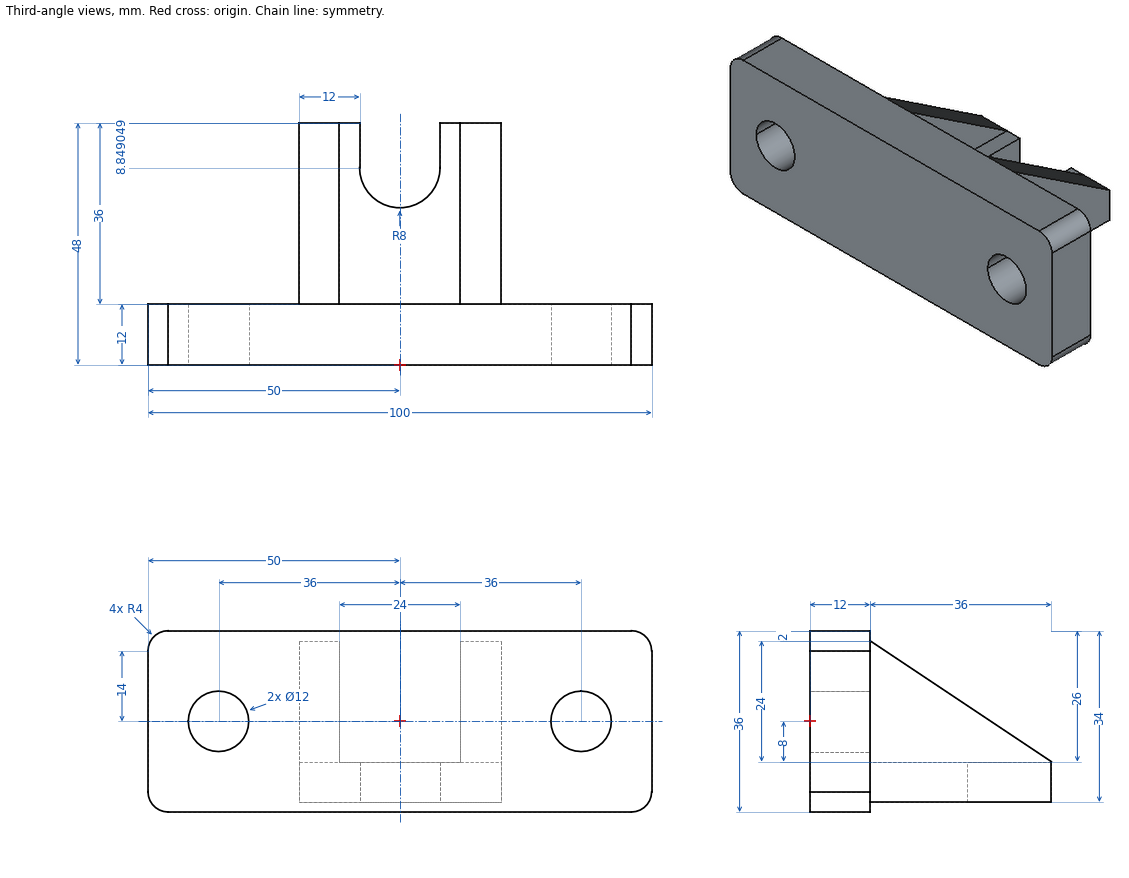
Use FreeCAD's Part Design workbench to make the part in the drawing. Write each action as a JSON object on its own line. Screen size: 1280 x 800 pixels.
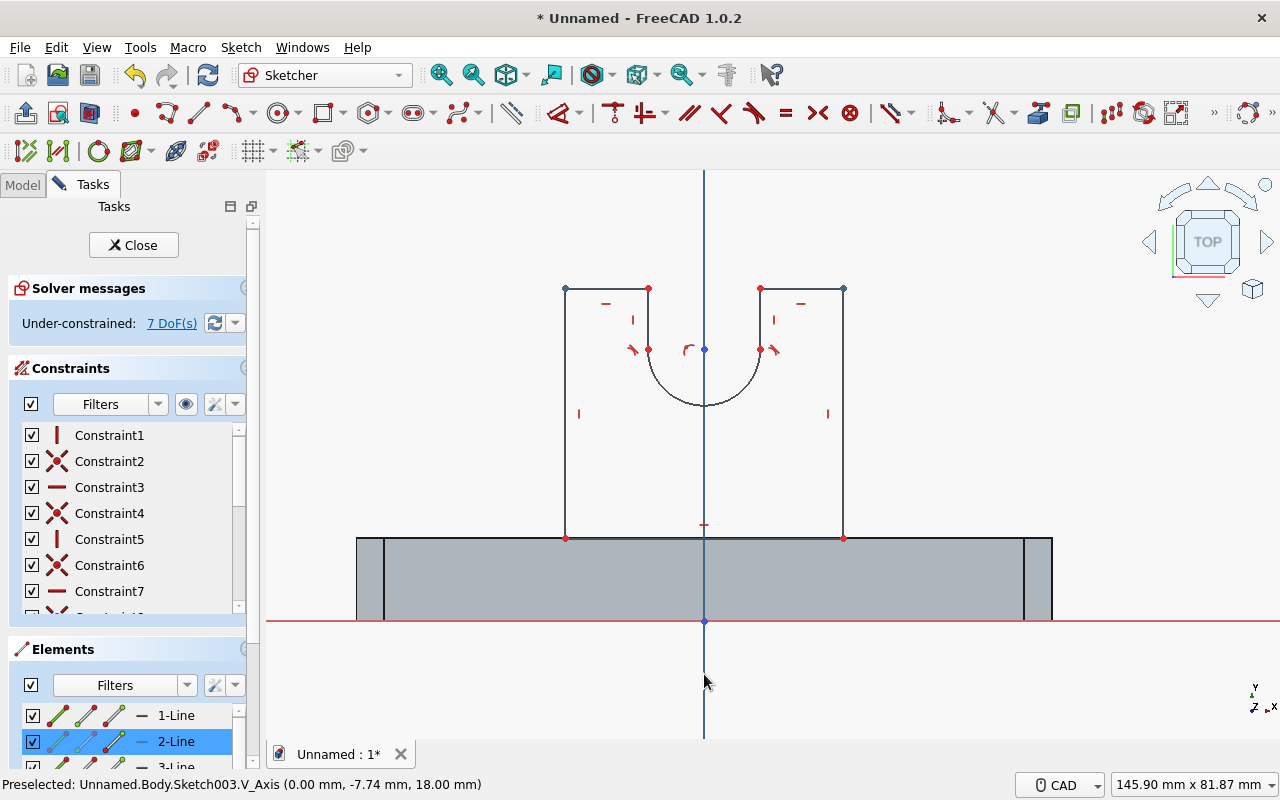
{"action": "left_click", "coordinate": [818, 114]}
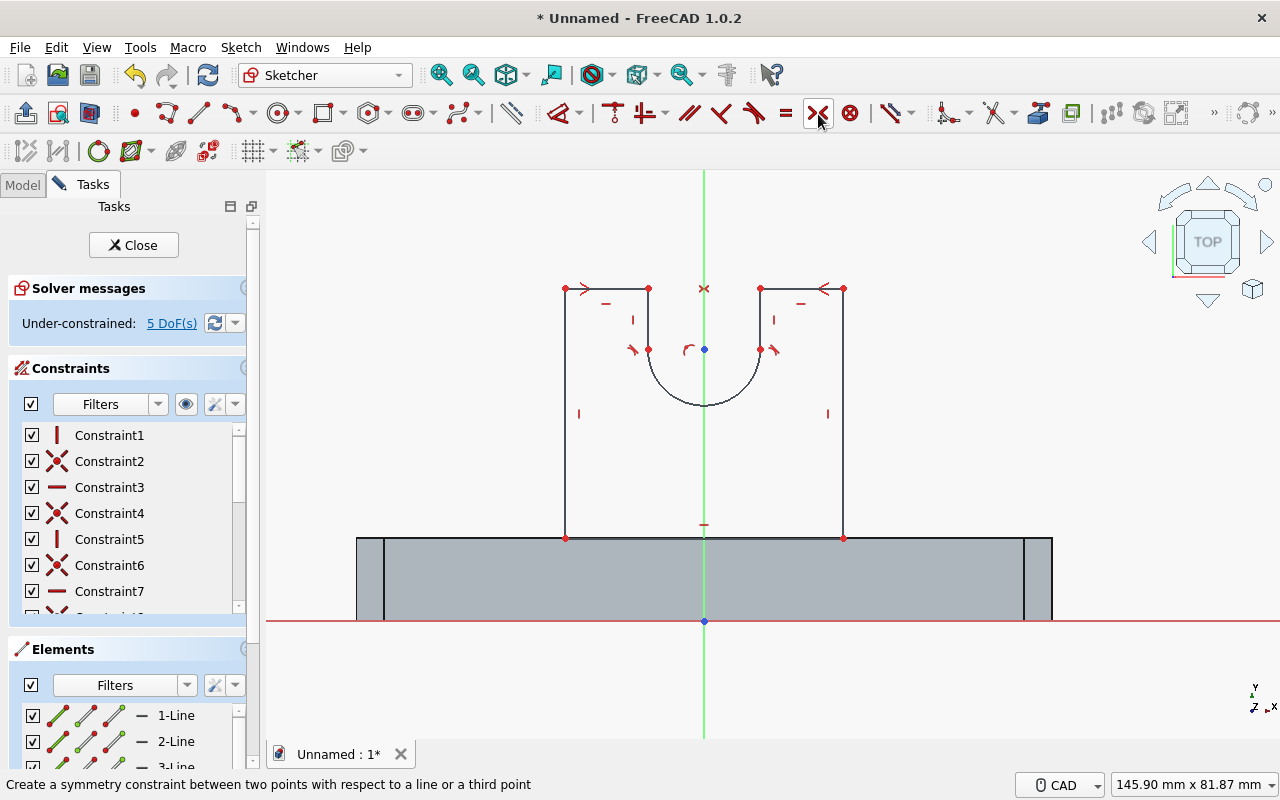
{"action": "left_click", "coordinate": [558, 114]}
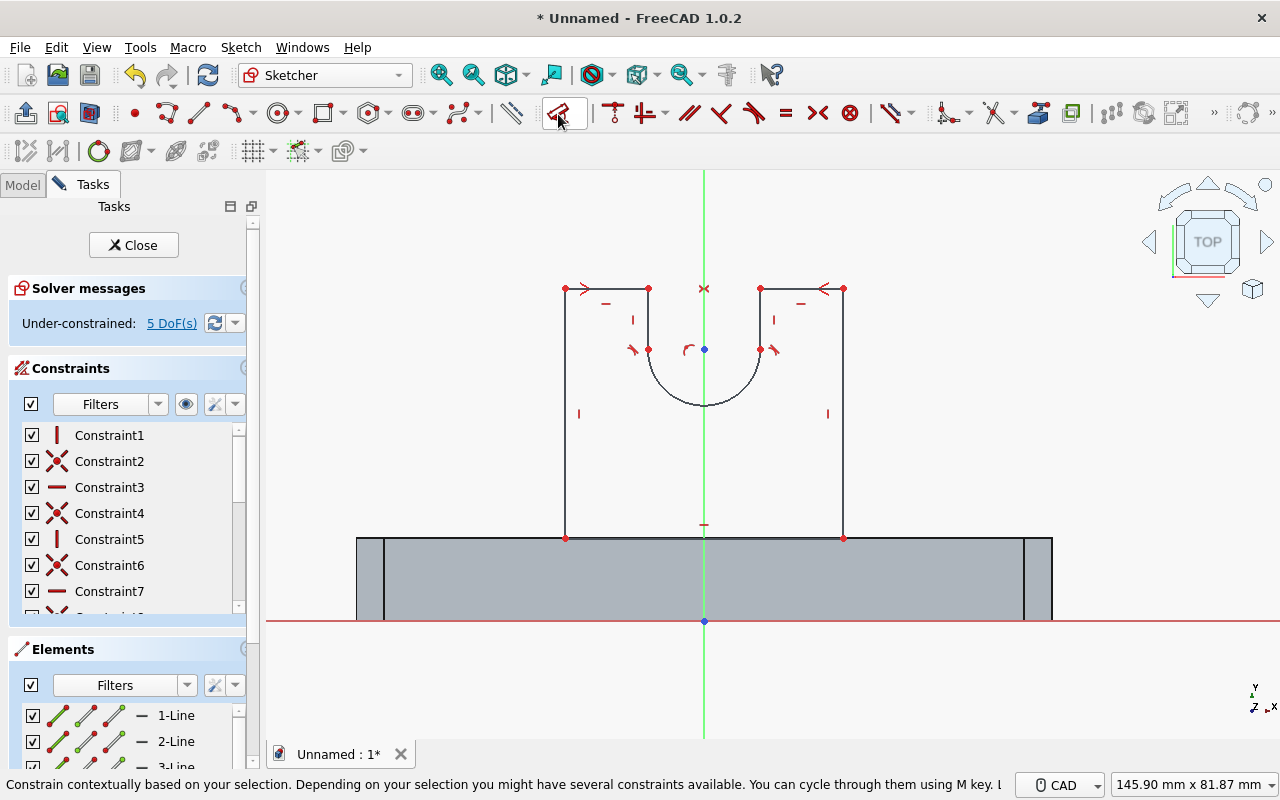
{"action": "left_click", "coordinate": [671, 395]}
{"action": "left_click", "coordinate": [652, 421]}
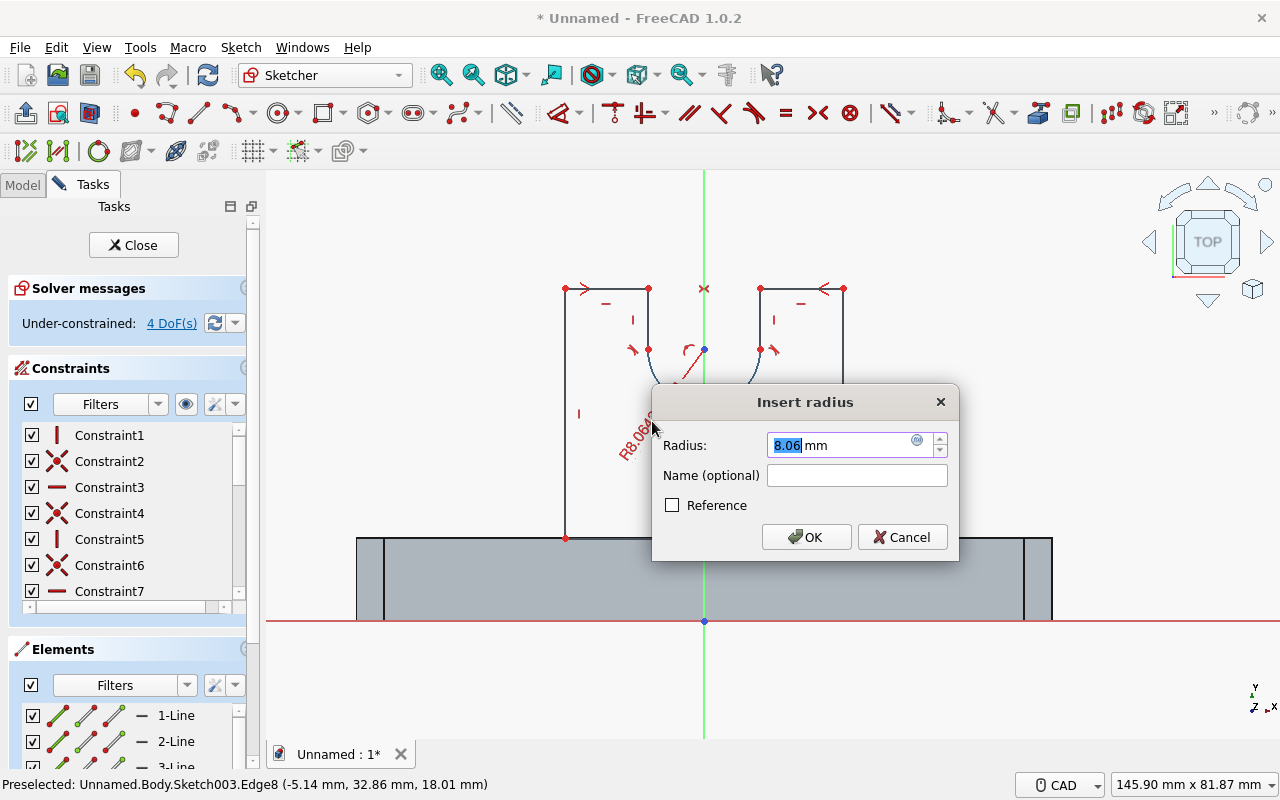
{"action": "type", "text": "8"}
{"action": "key", "text": "Return"}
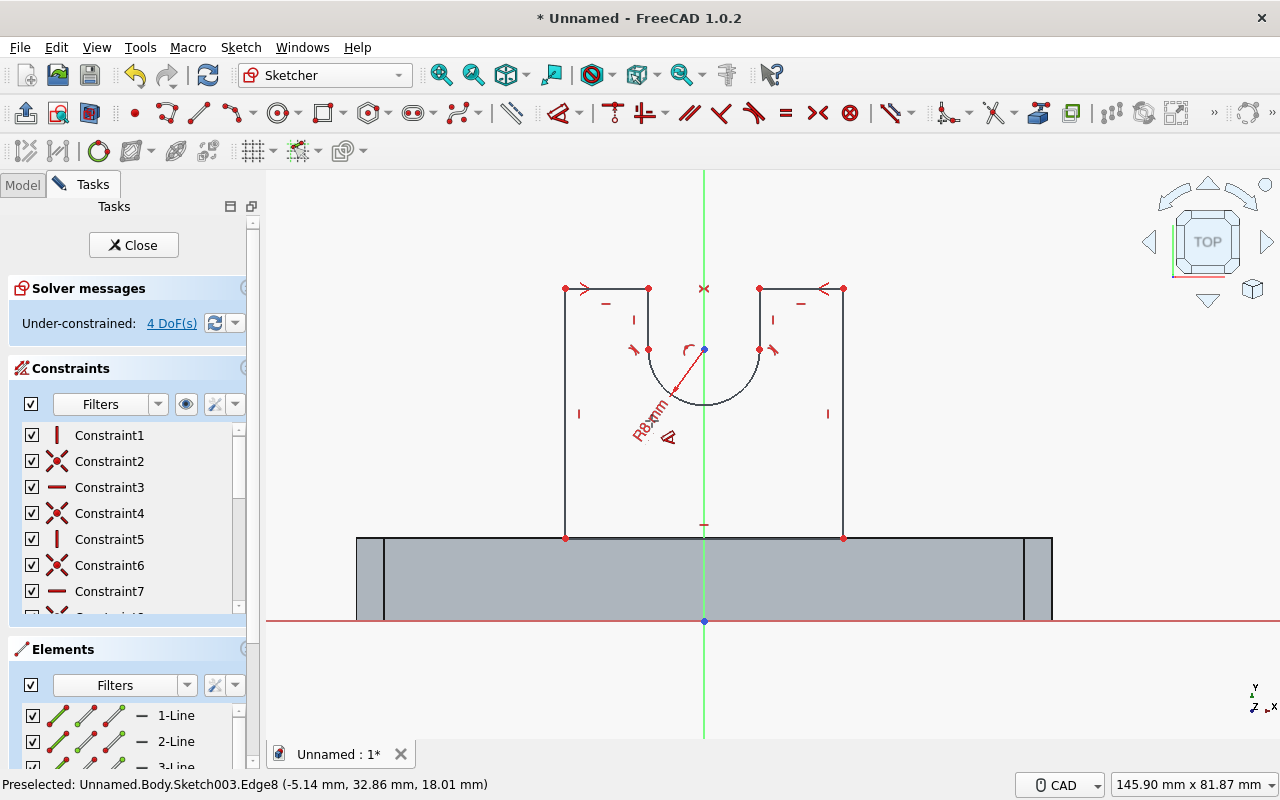
{"action": "left_click", "coordinate": [623, 289]}
{"action": "left_click", "coordinate": [607, 255]}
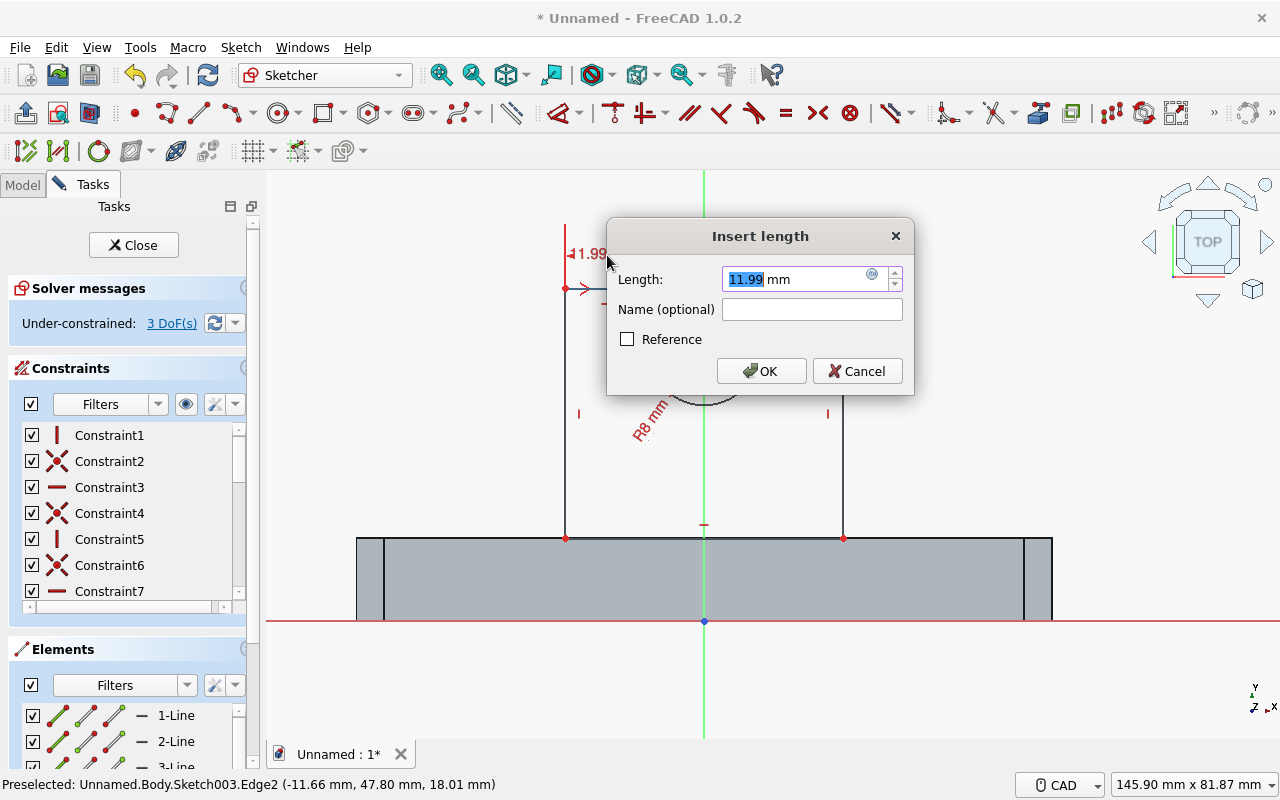
{"action": "type", "text": "12"}
{"action": "key", "text": "Return"}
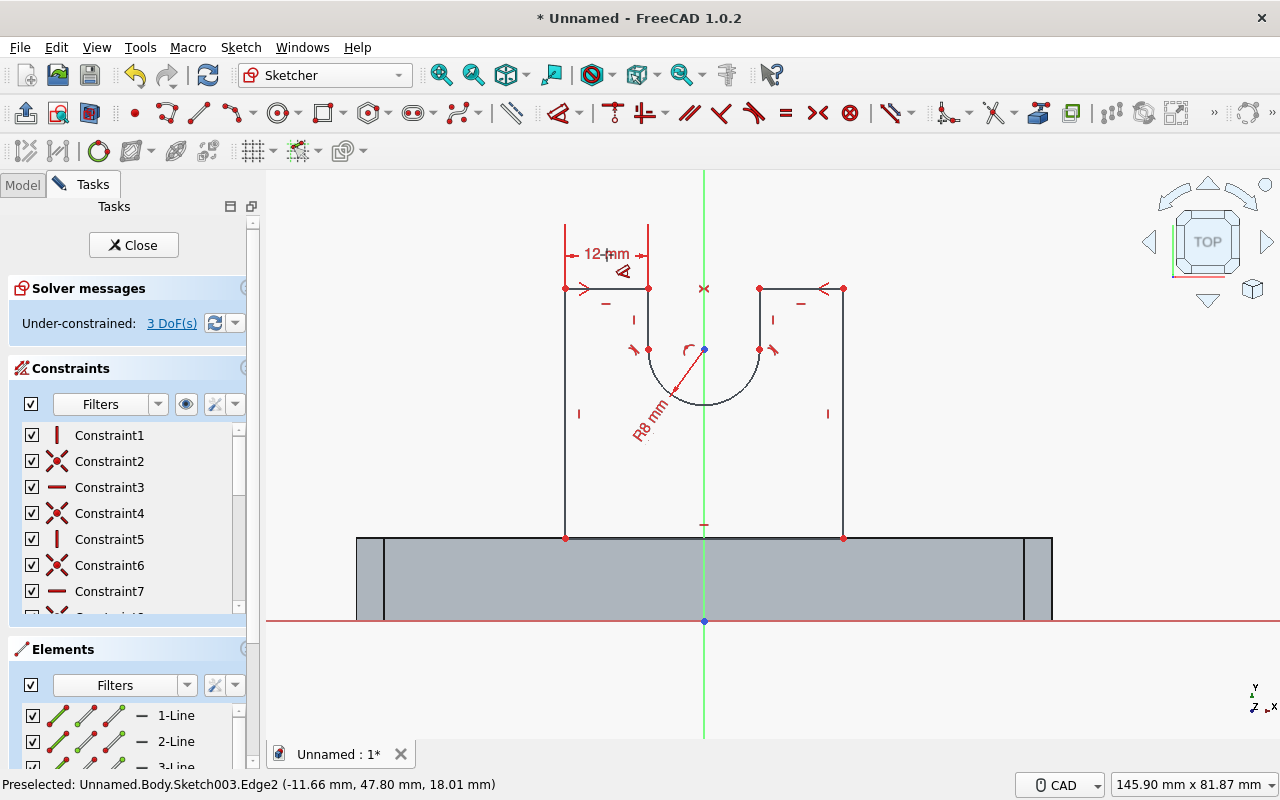
{"action": "left_click", "coordinate": [565, 364]}
{"action": "left_click", "coordinate": [531, 414]}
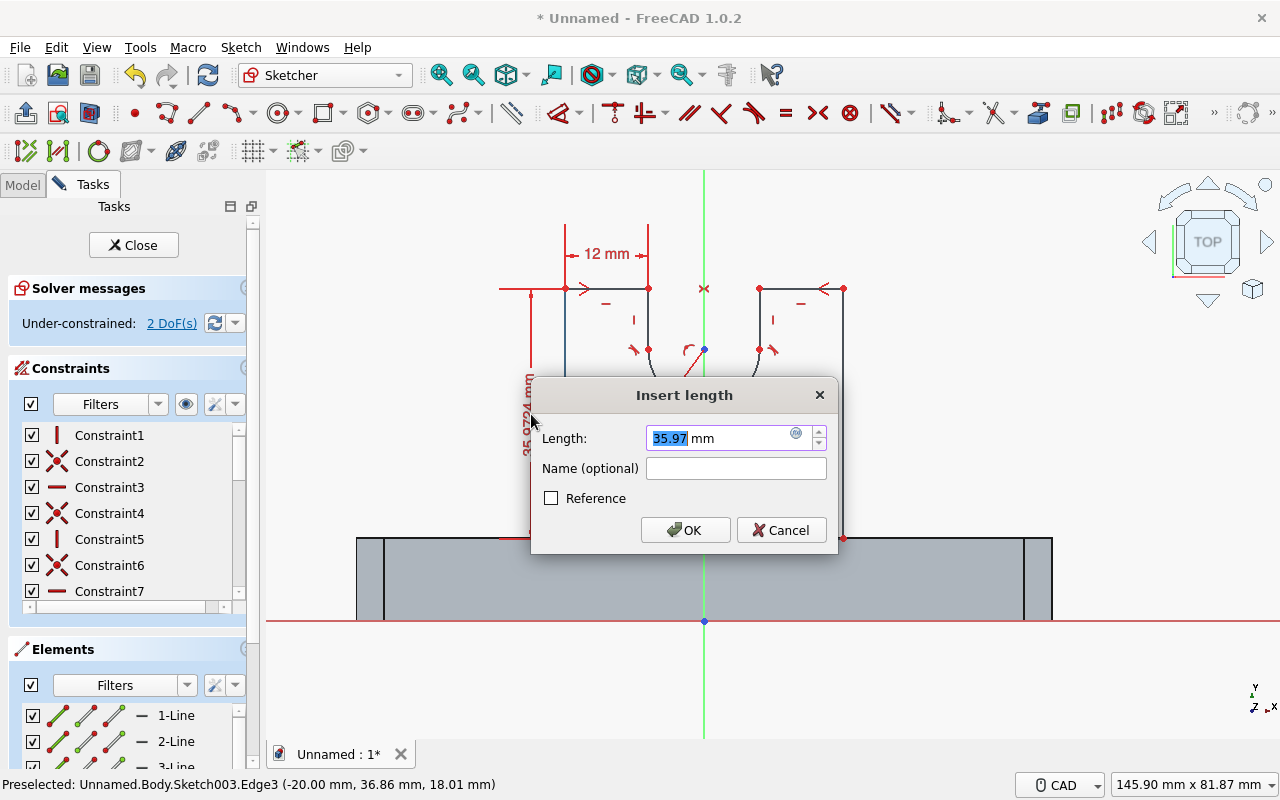
{"action": "type", "text": "36"}
{"action": "key", "text": "Return"}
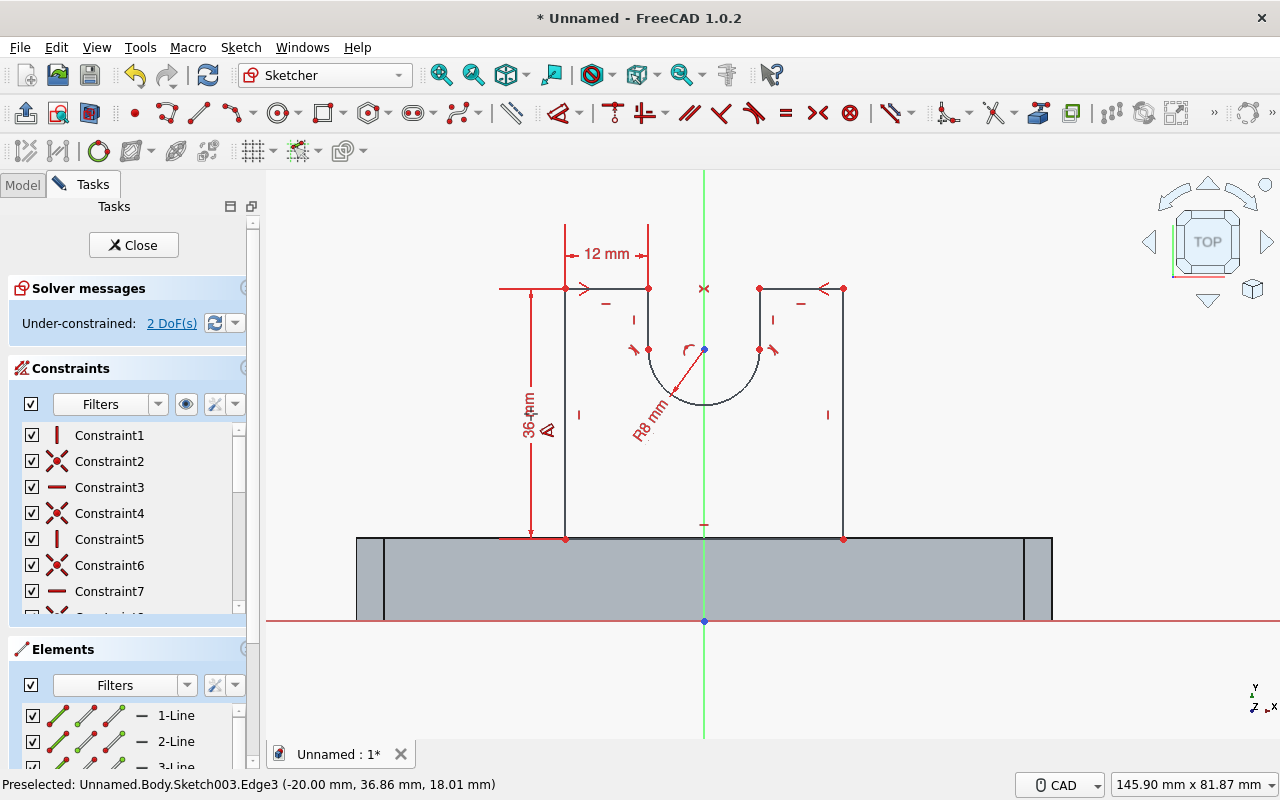
{"action": "left_click", "coordinate": [648, 289]}
{"action": "left_click", "coordinate": [614, 455]}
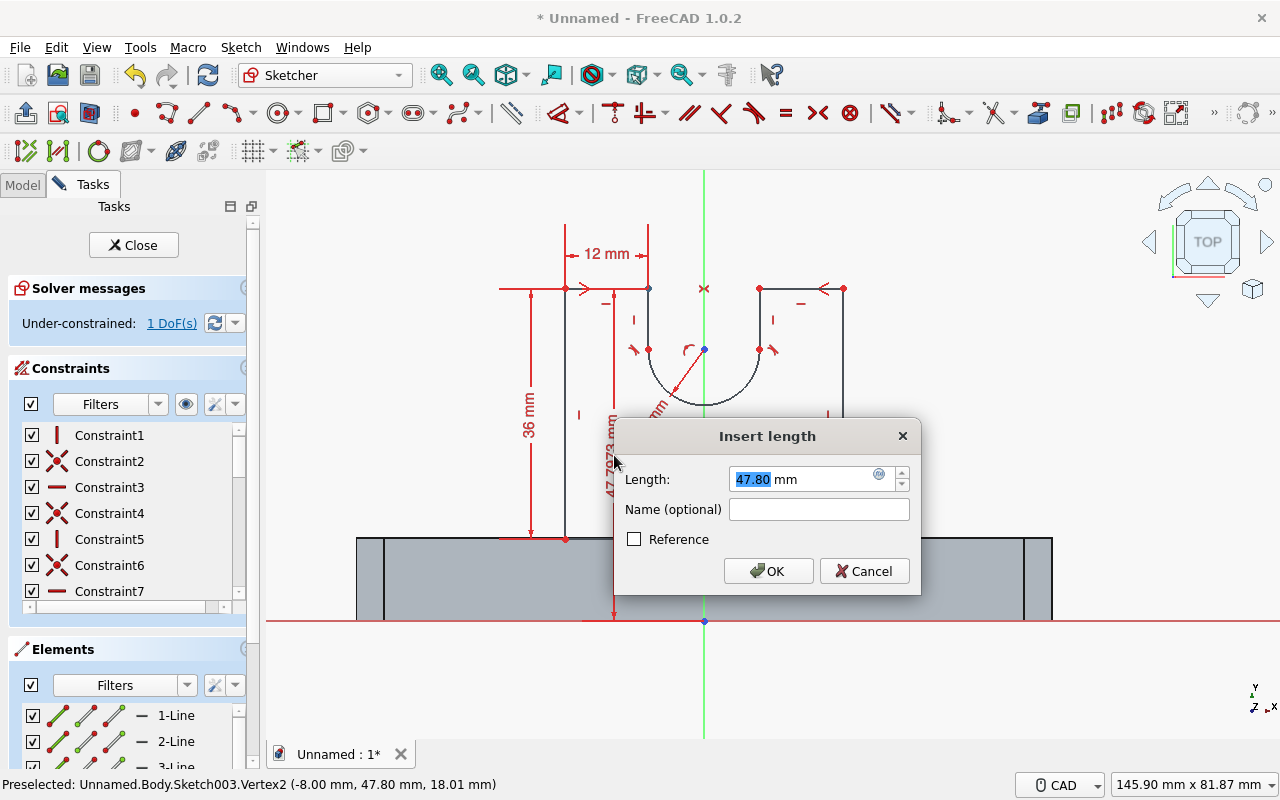
{"action": "type", "text": "48"}
{"action": "key", "text": "Return"}